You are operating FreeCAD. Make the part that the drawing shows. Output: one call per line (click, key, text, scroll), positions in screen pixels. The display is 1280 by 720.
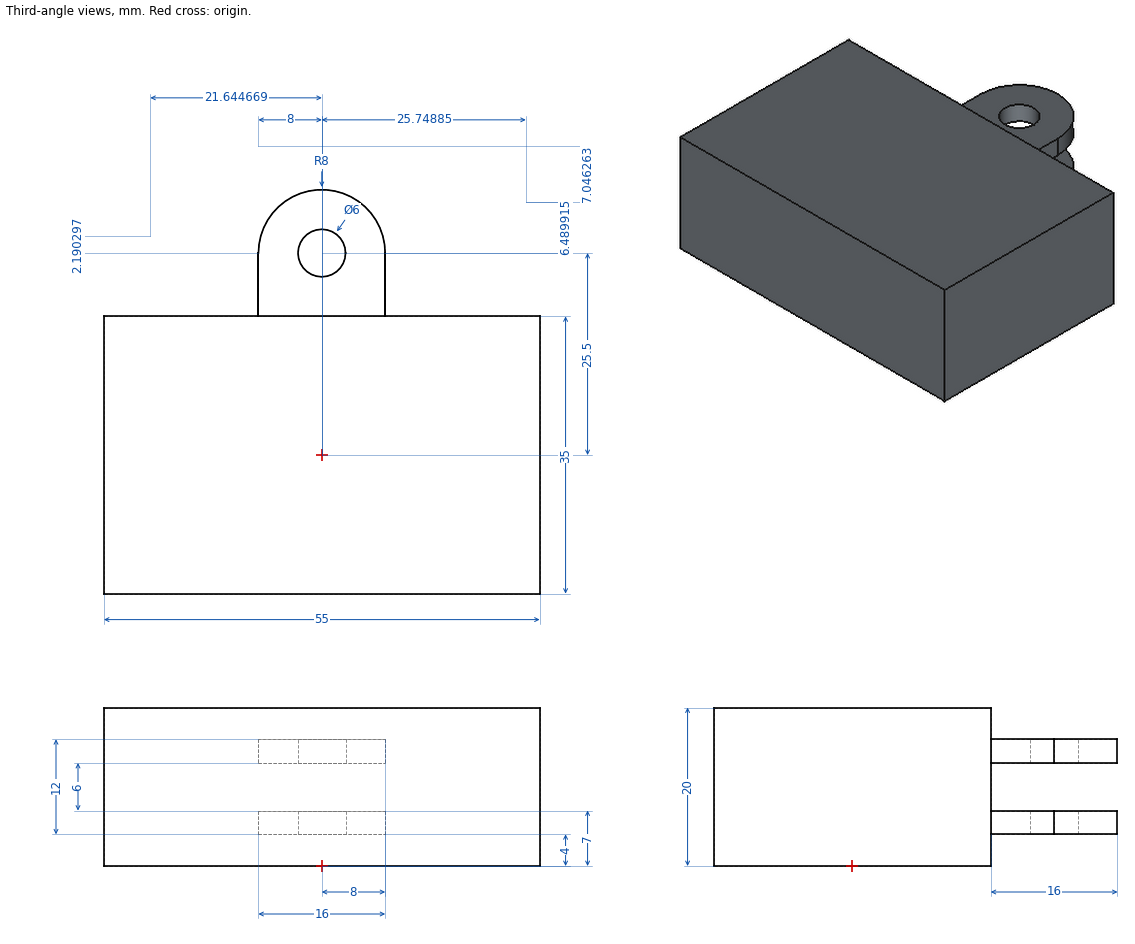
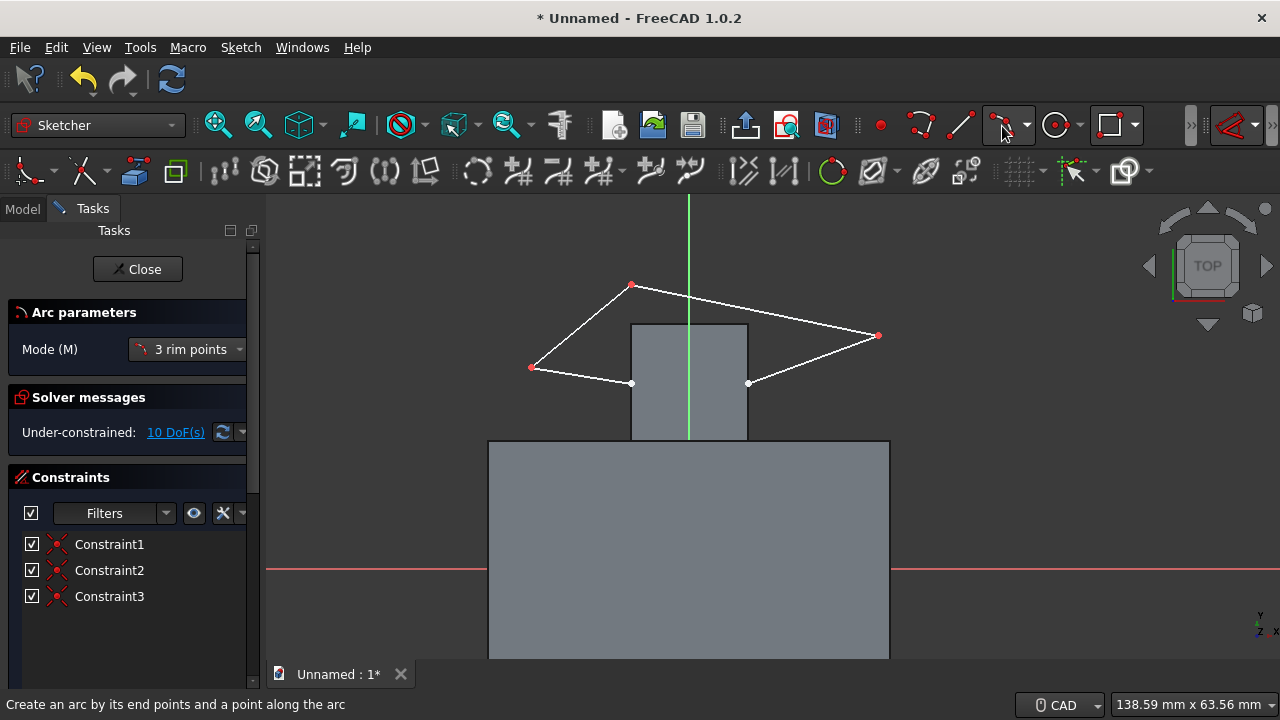
click(631, 384)
click(748, 384)
click(707, 327)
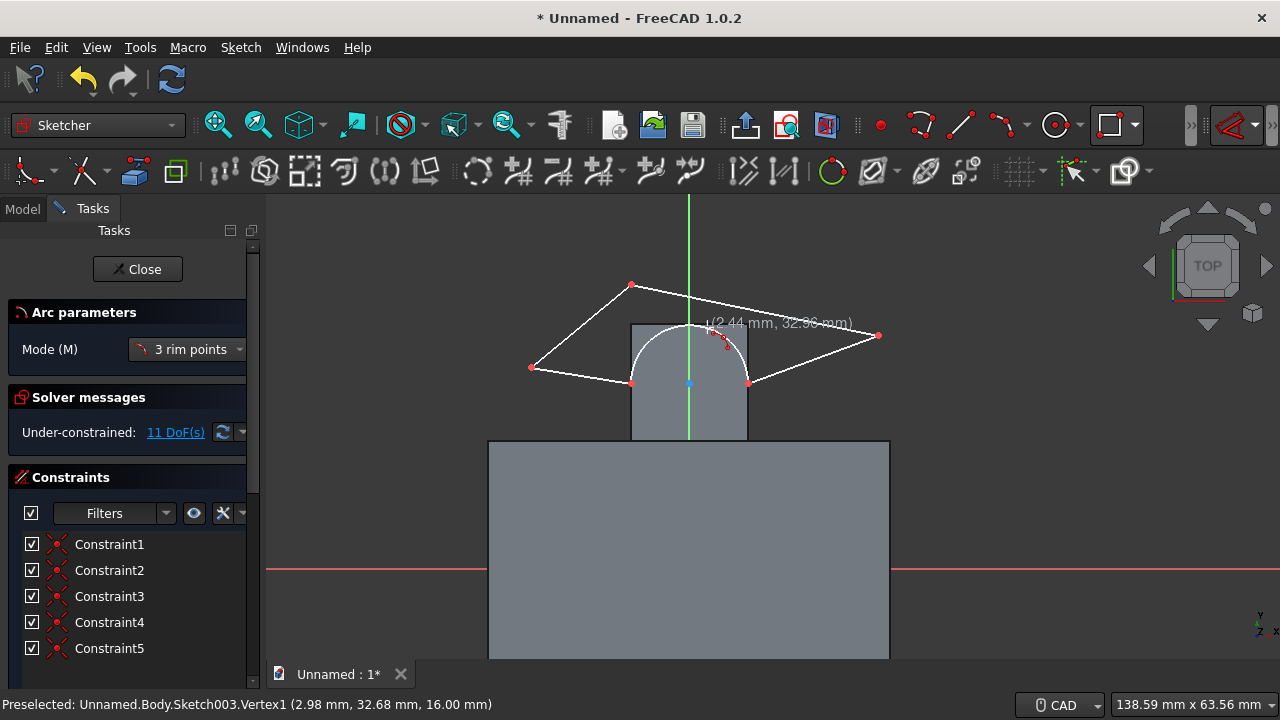
click(1056, 126)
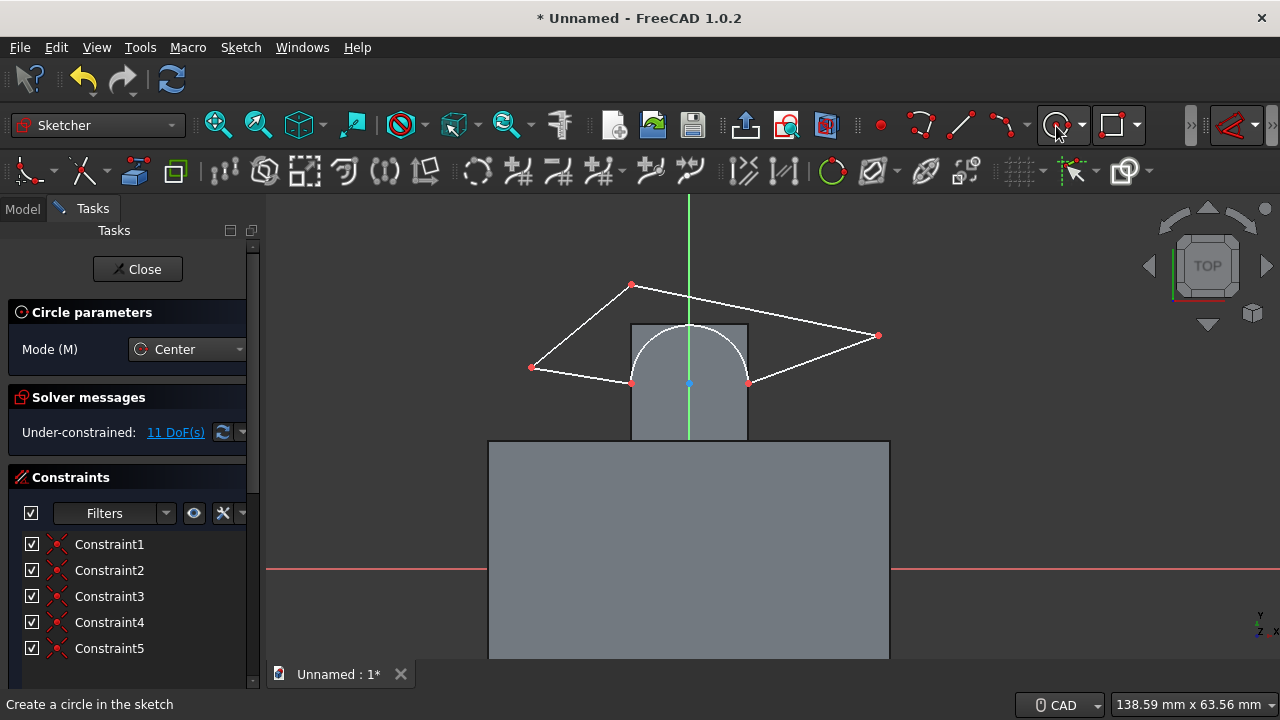
click(689, 383)
move(705, 367)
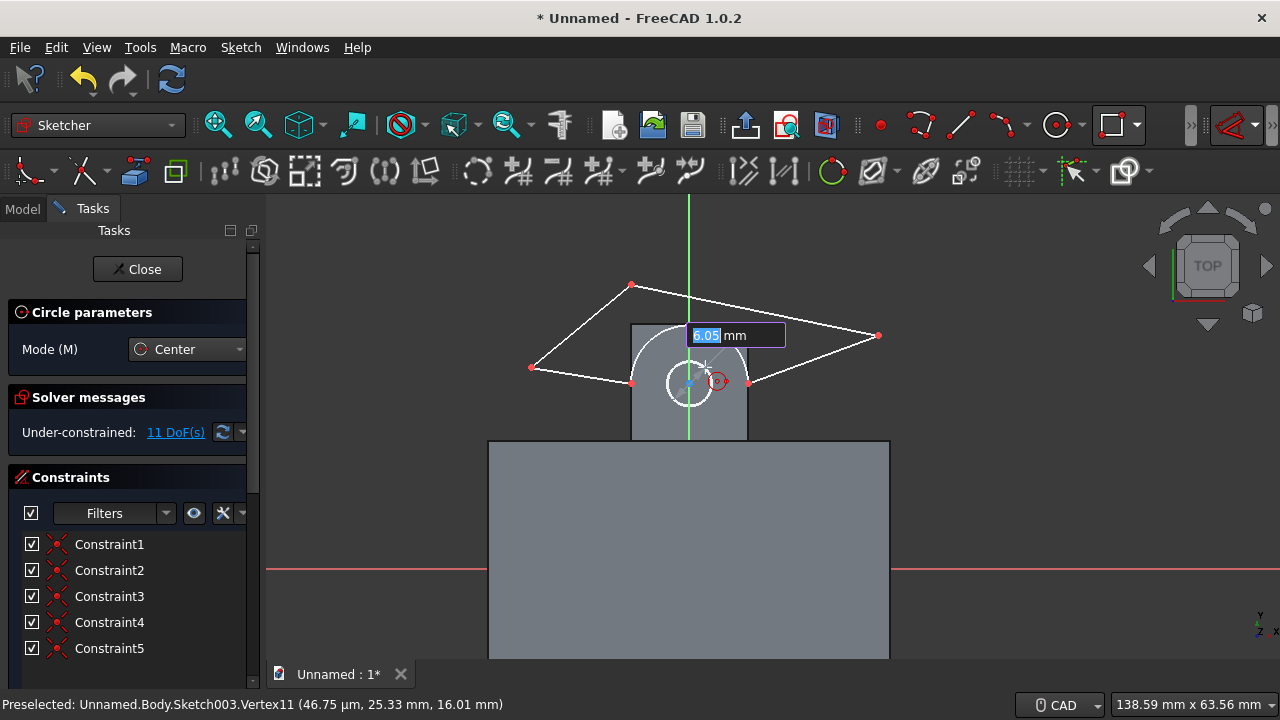
text(6)
key(Return)
key(Escape)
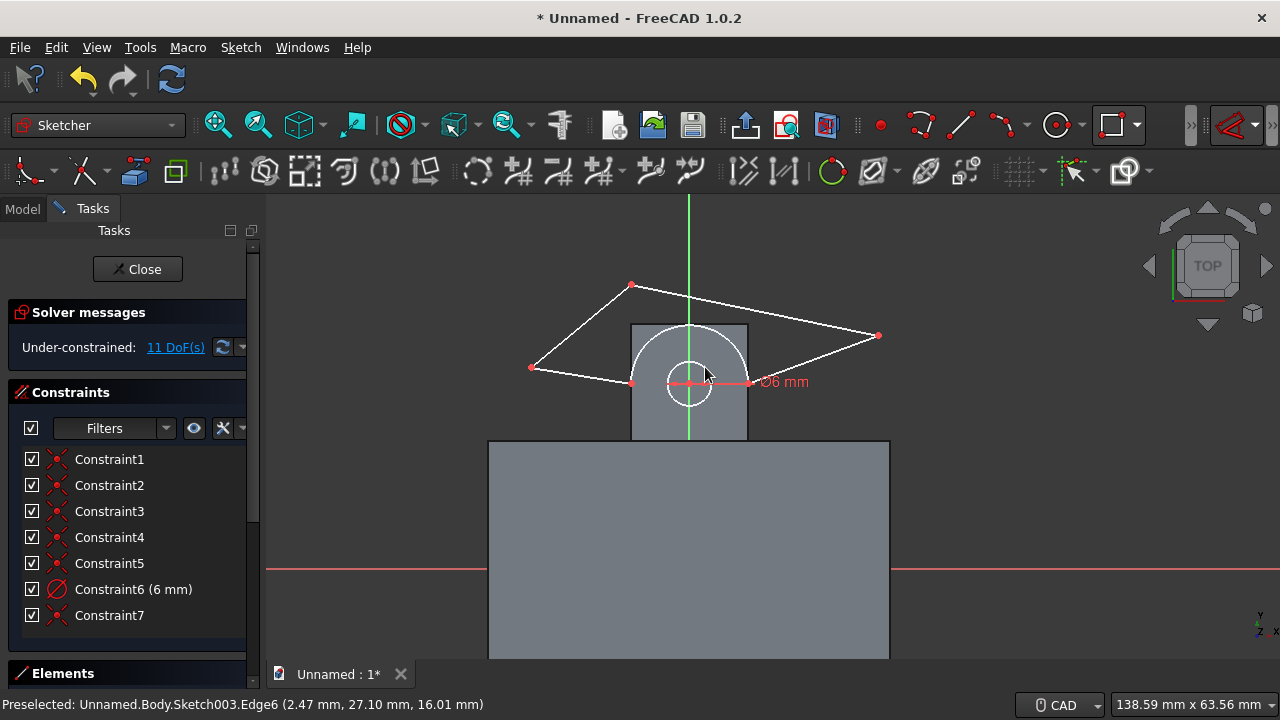
click(689, 384)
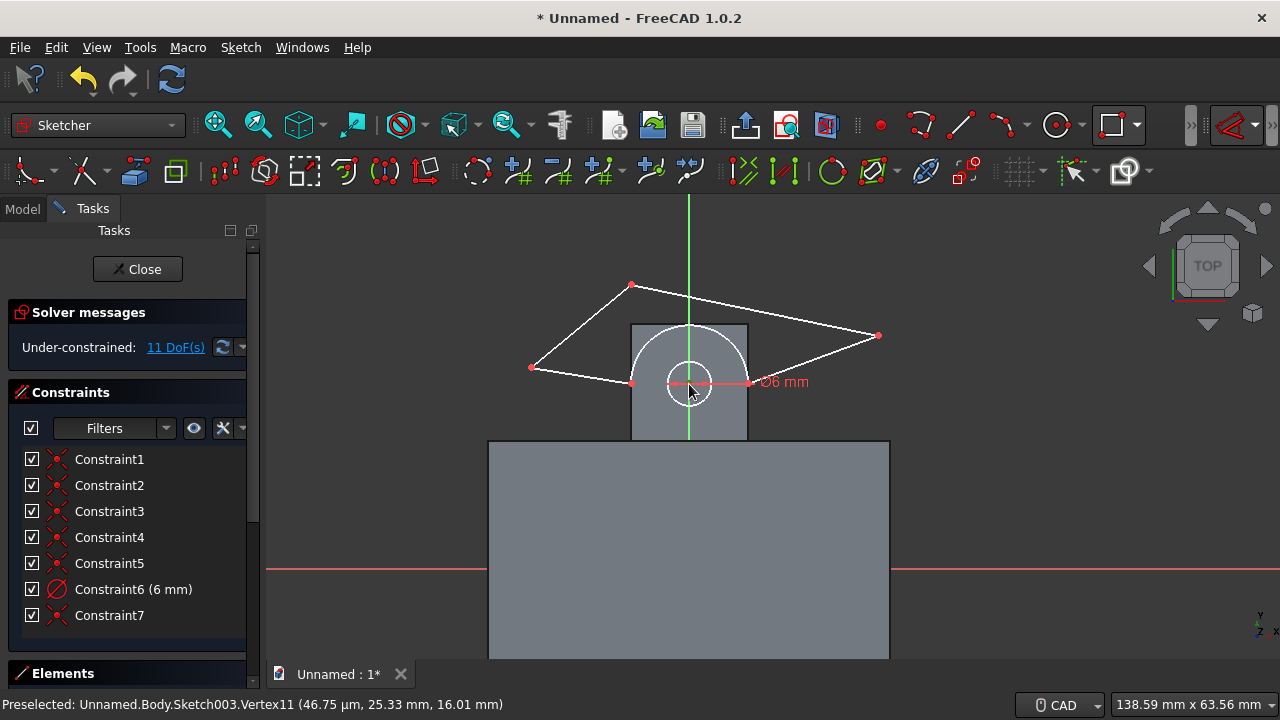
click(689, 602)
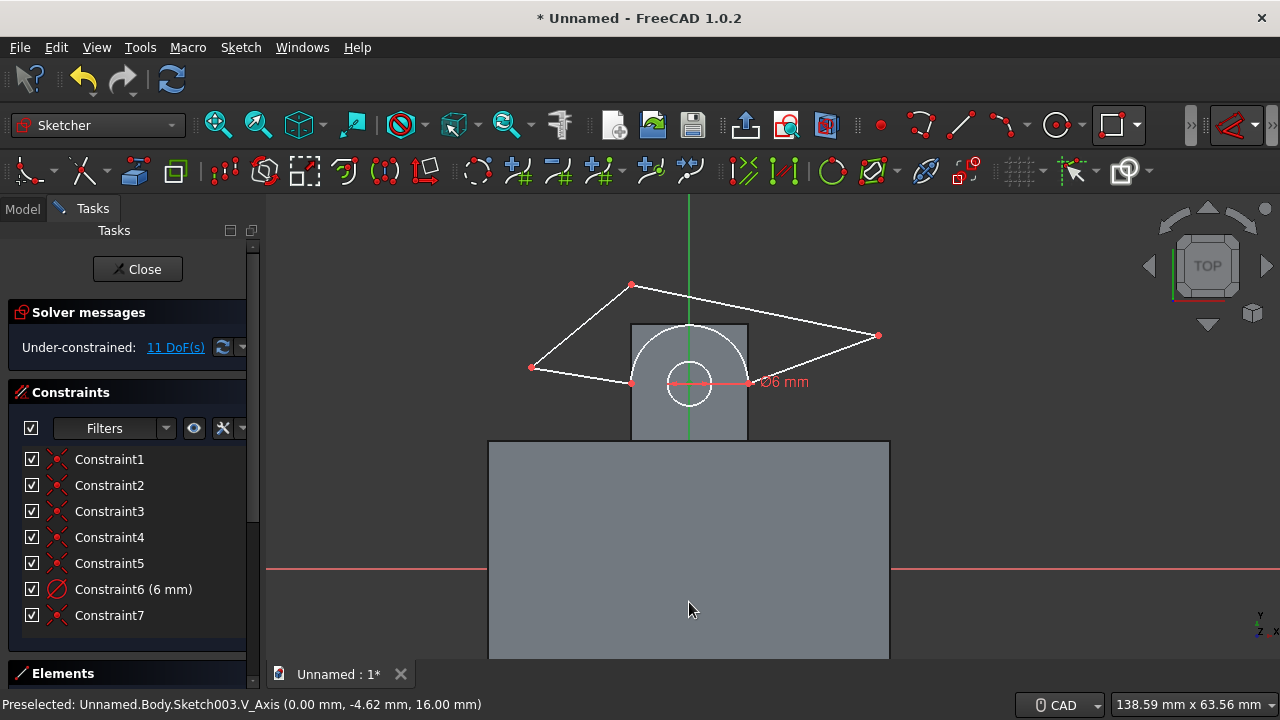
key(c)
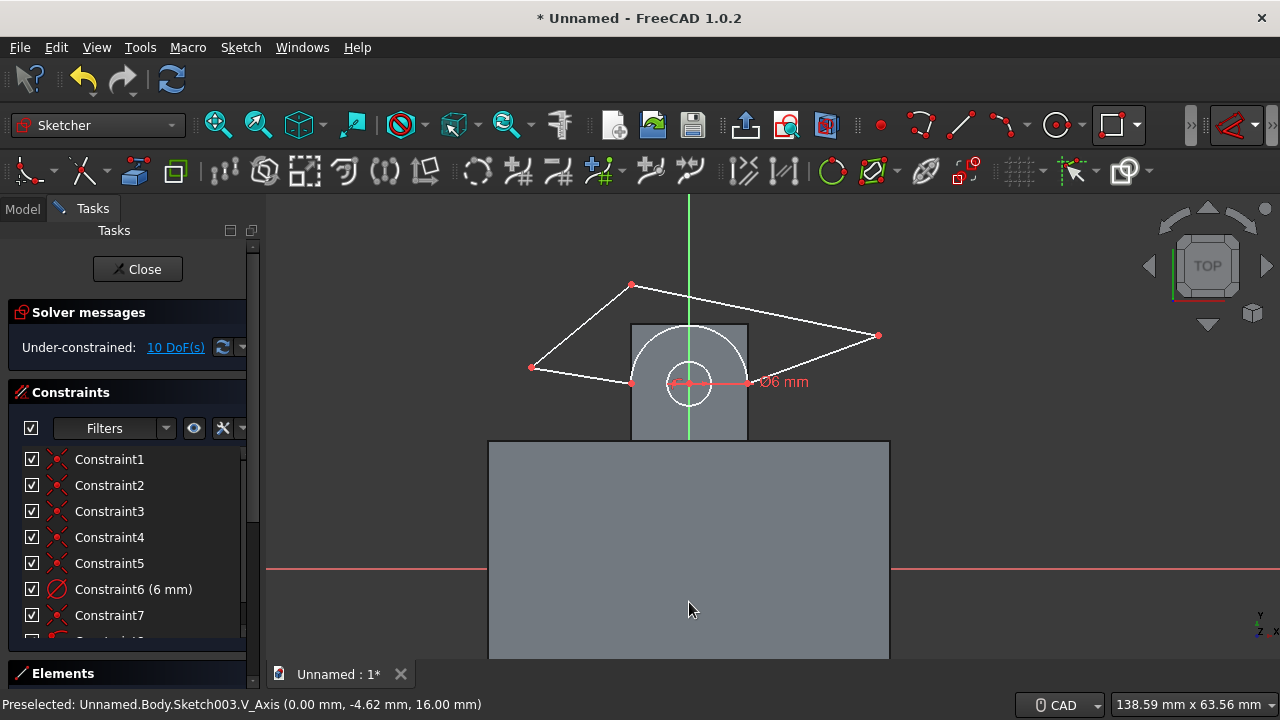
click(723, 337)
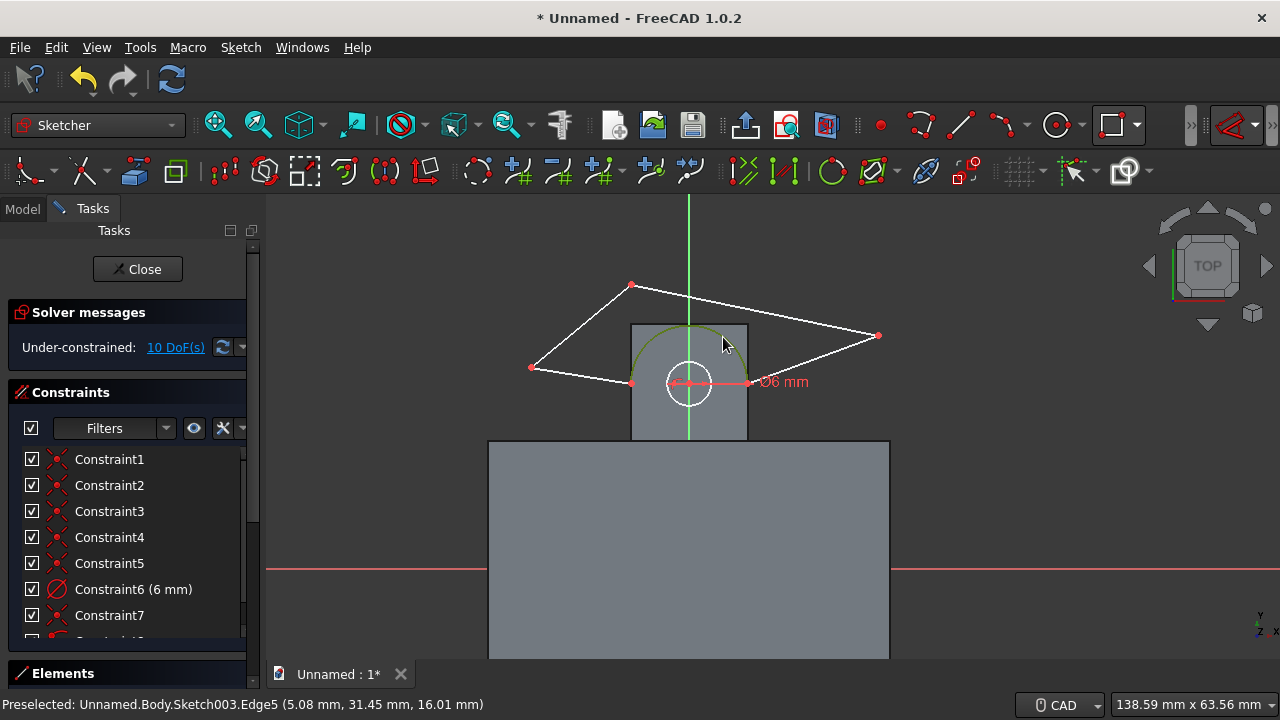
key(k)
key(r)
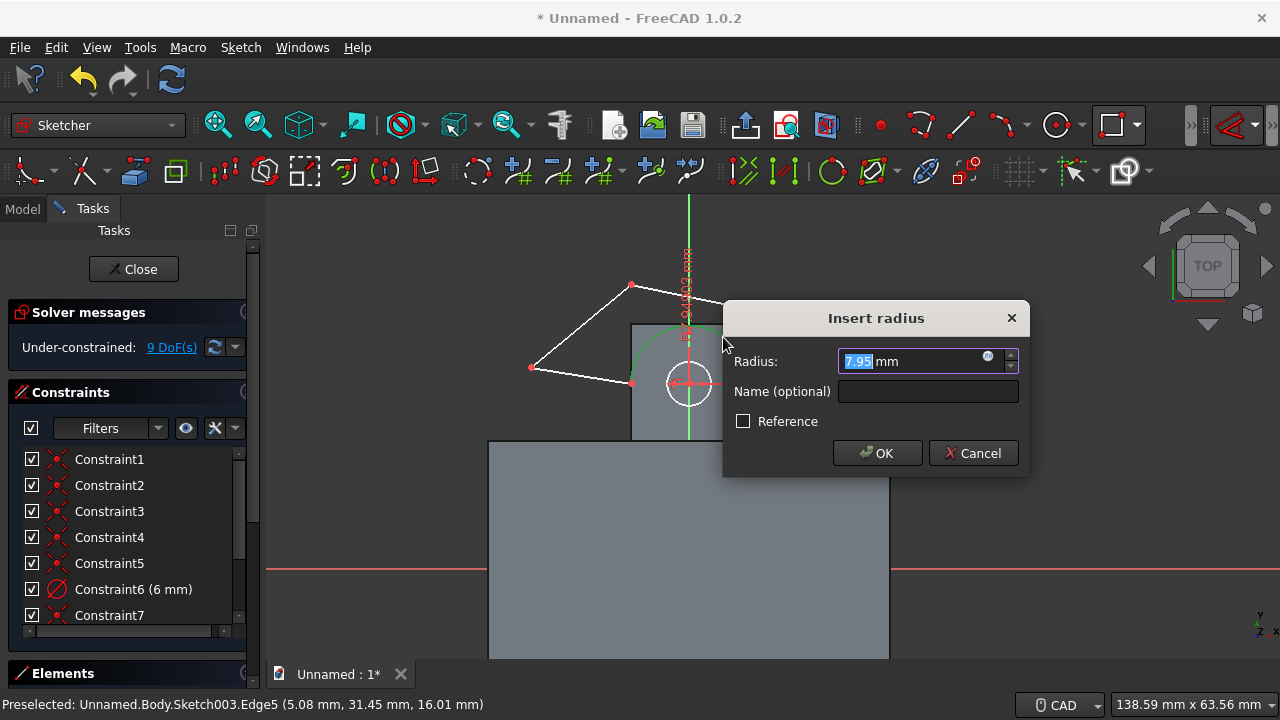
text(8)
key(Return)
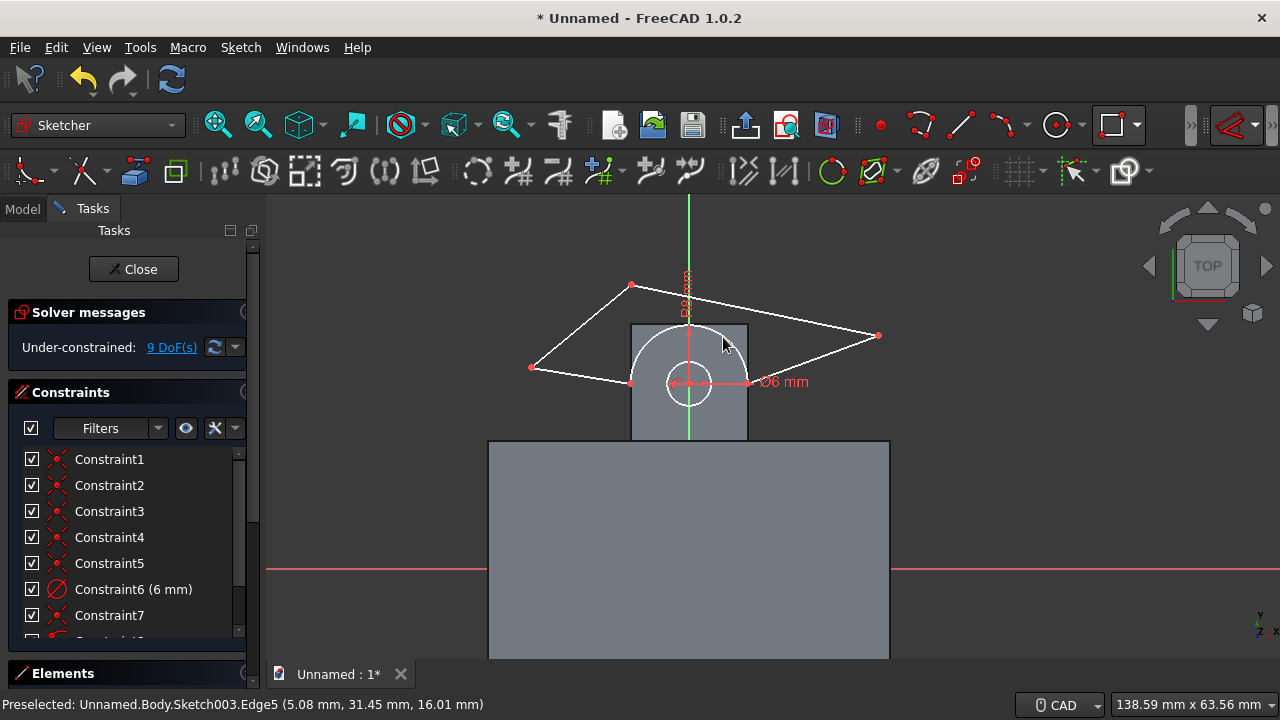
click(631, 285)